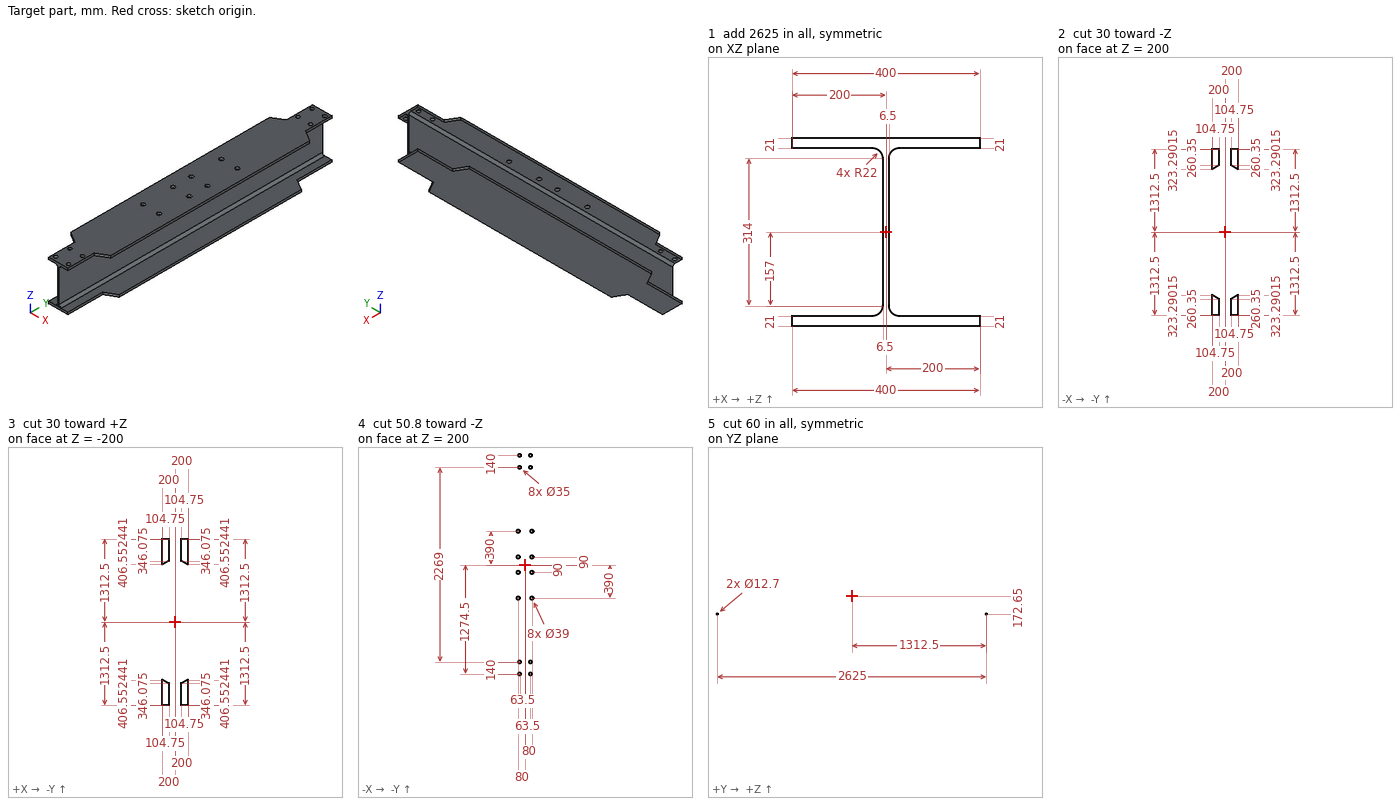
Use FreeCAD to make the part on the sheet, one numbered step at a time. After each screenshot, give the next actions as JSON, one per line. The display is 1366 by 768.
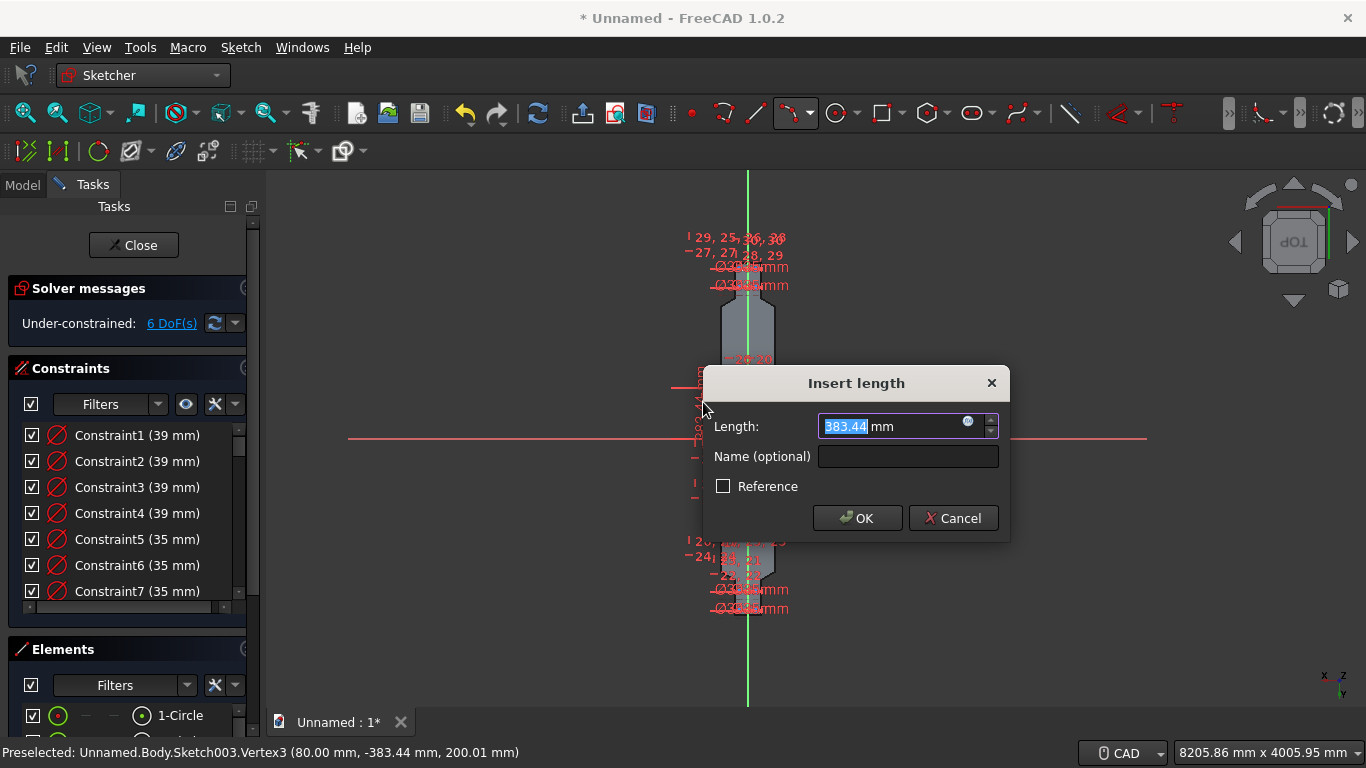
{"action": "type", "text": "390"}
{"action": "key", "text": "Return"}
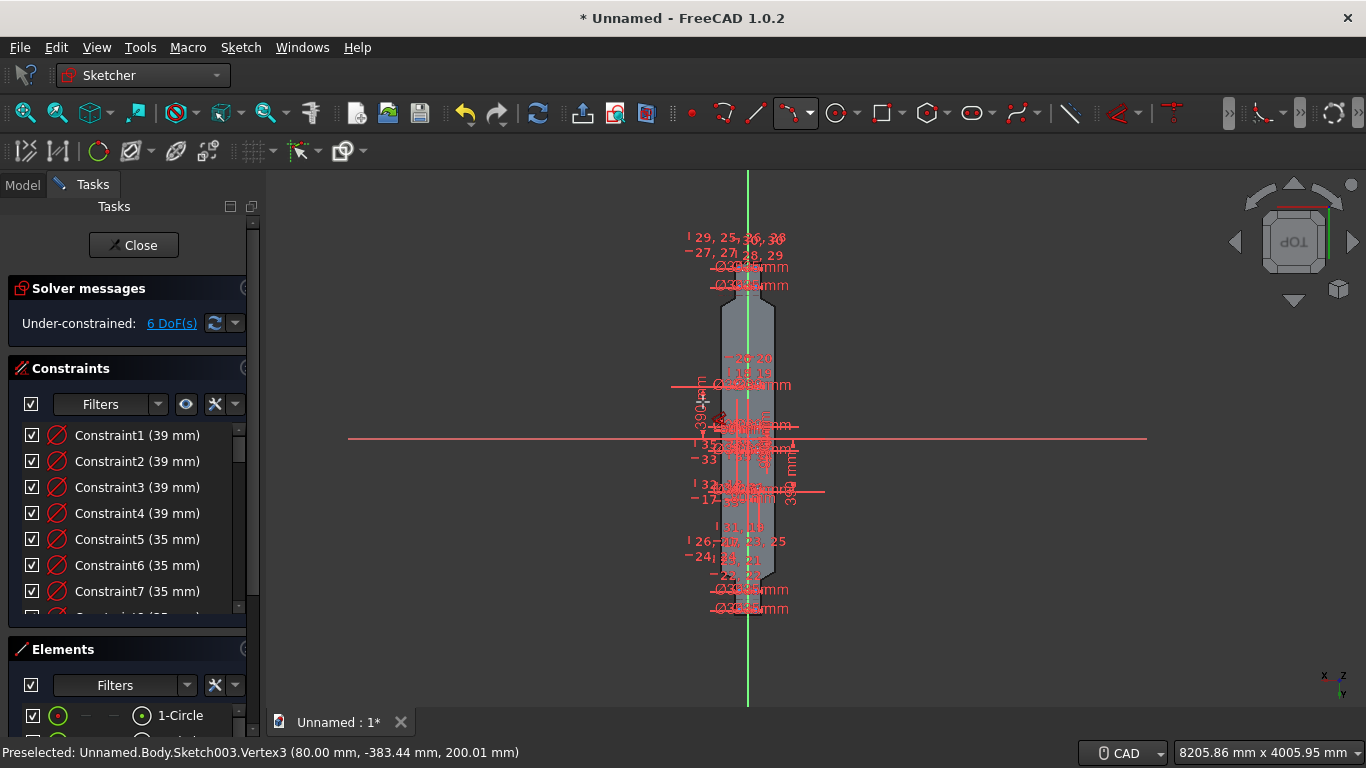
{"action": "scroll", "coordinate": [740, 611], "scroll_direction": "up", "scroll_amount": 8}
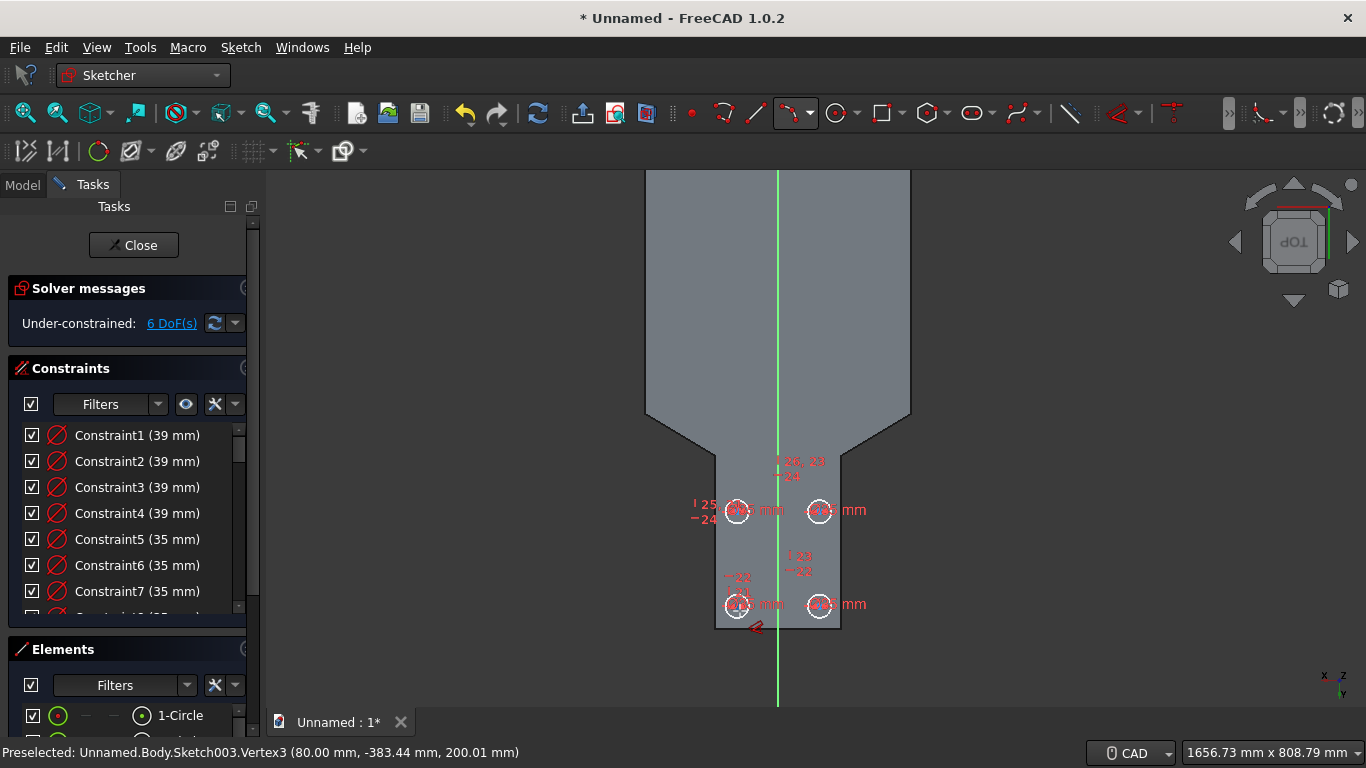
{"action": "left_click", "coordinate": [737, 606]}
{"action": "left_click", "coordinate": [758, 640]}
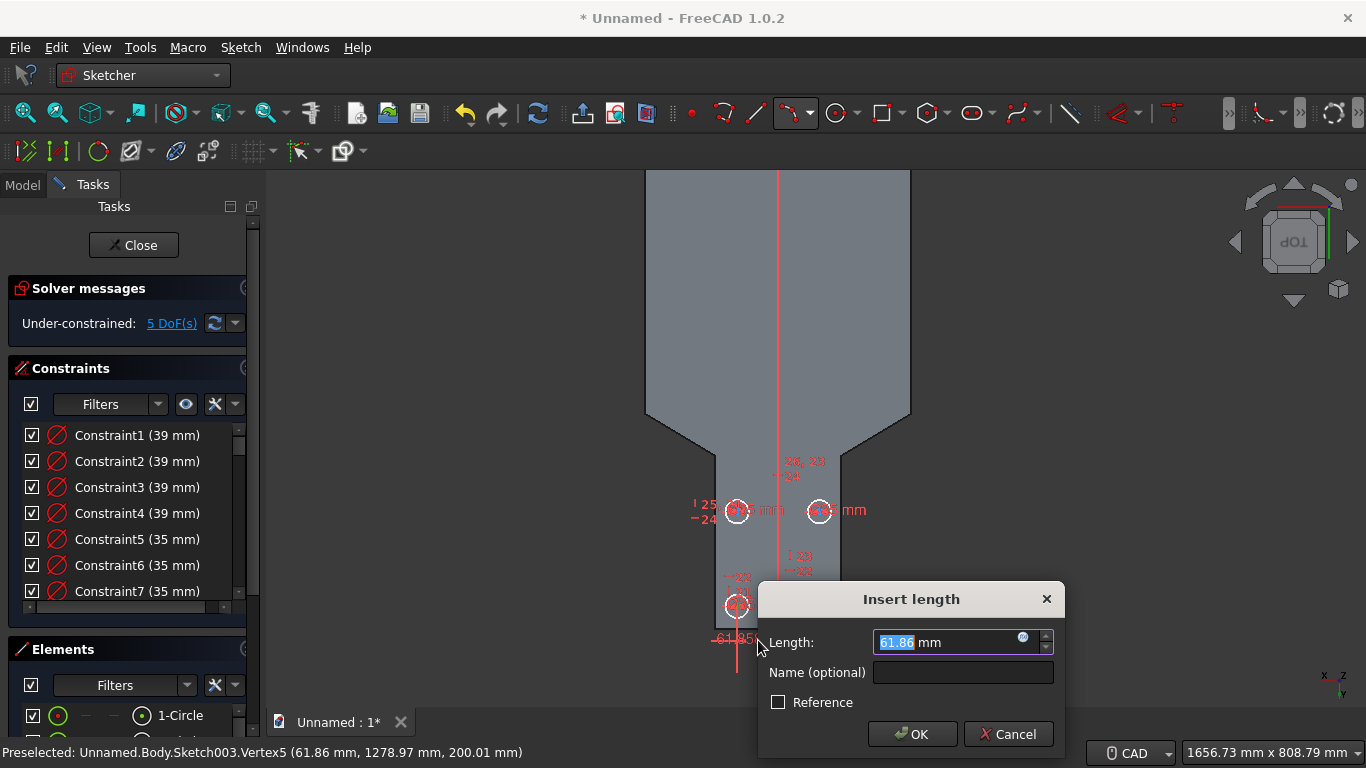
{"action": "type", "text": "63.5"}
{"action": "key", "text": "Return"}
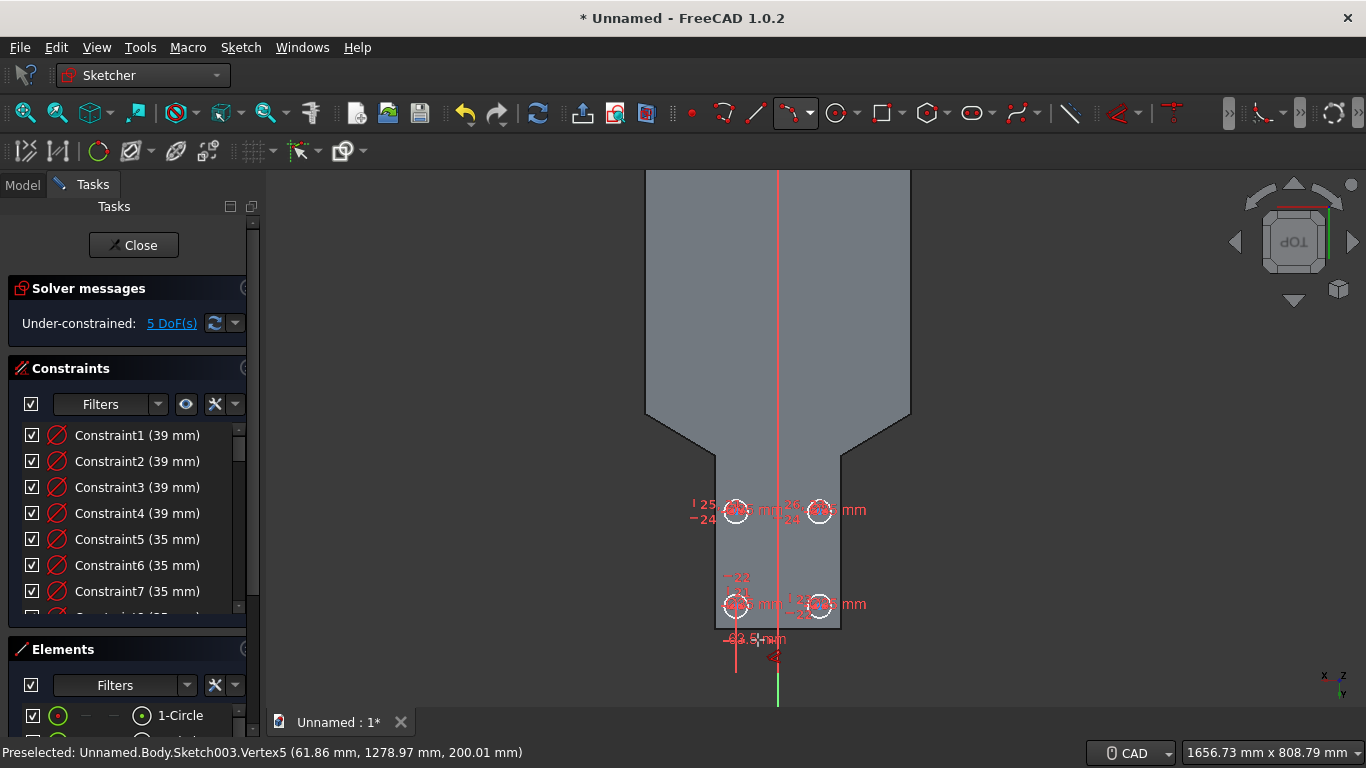
{"action": "left_click", "coordinate": [820, 606]}
{"action": "left_click", "coordinate": [799, 664]}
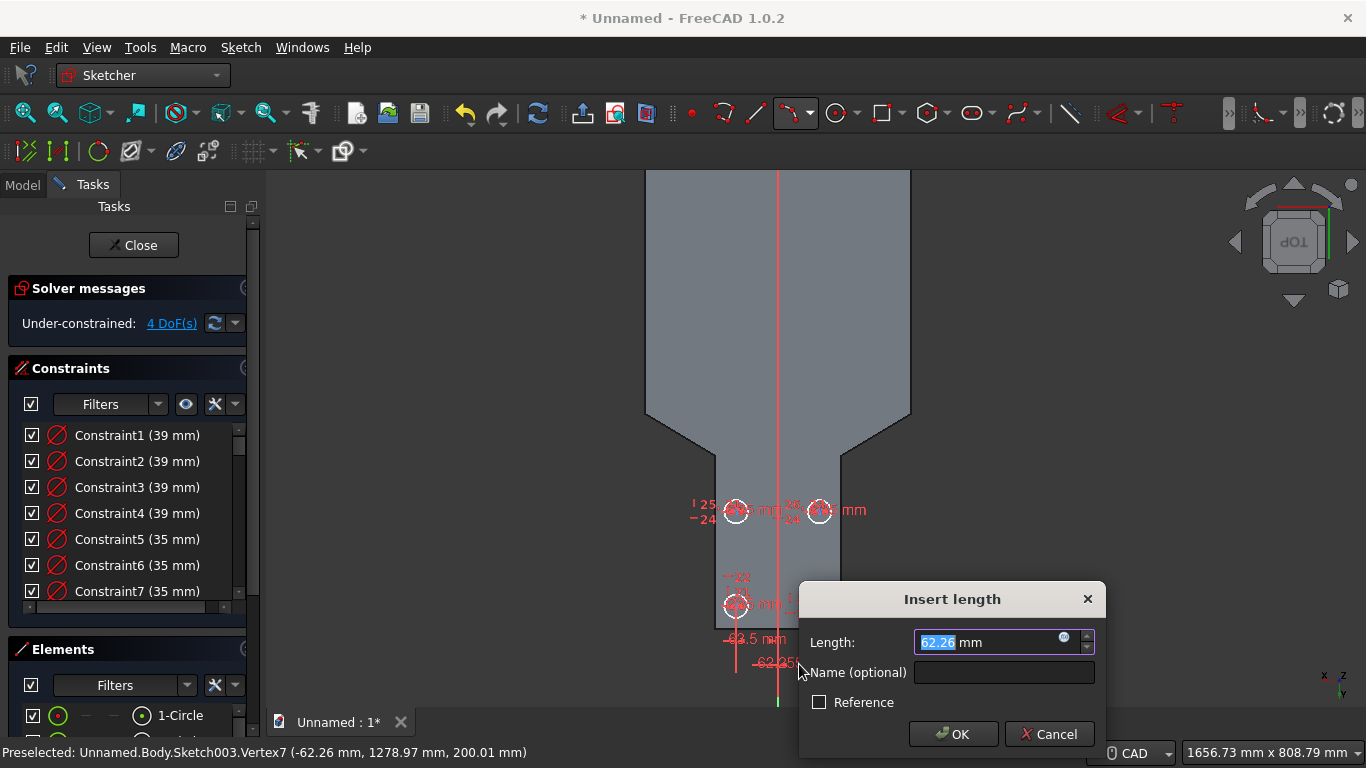
{"action": "type", "text": "63.5"}
{"action": "key", "text": "Return"}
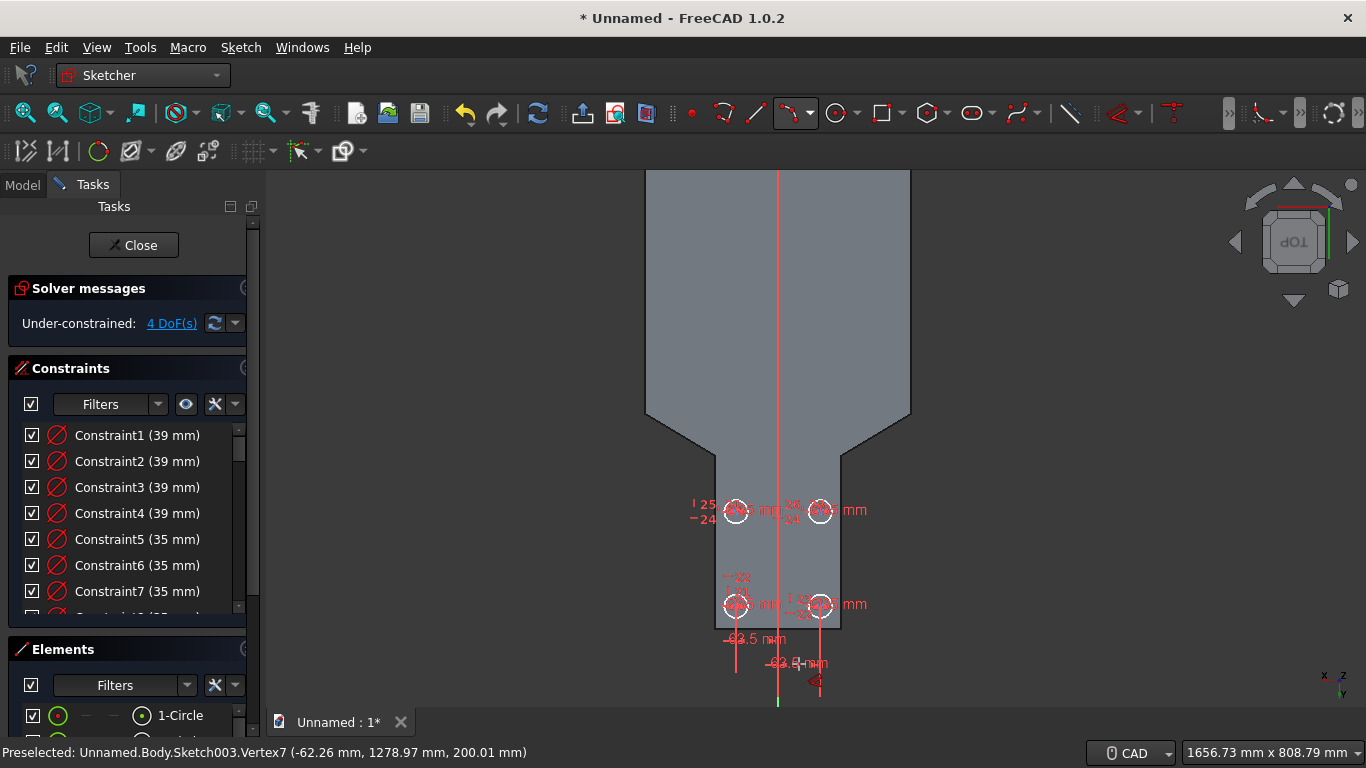
{"action": "left_click", "coordinate": [736, 606]}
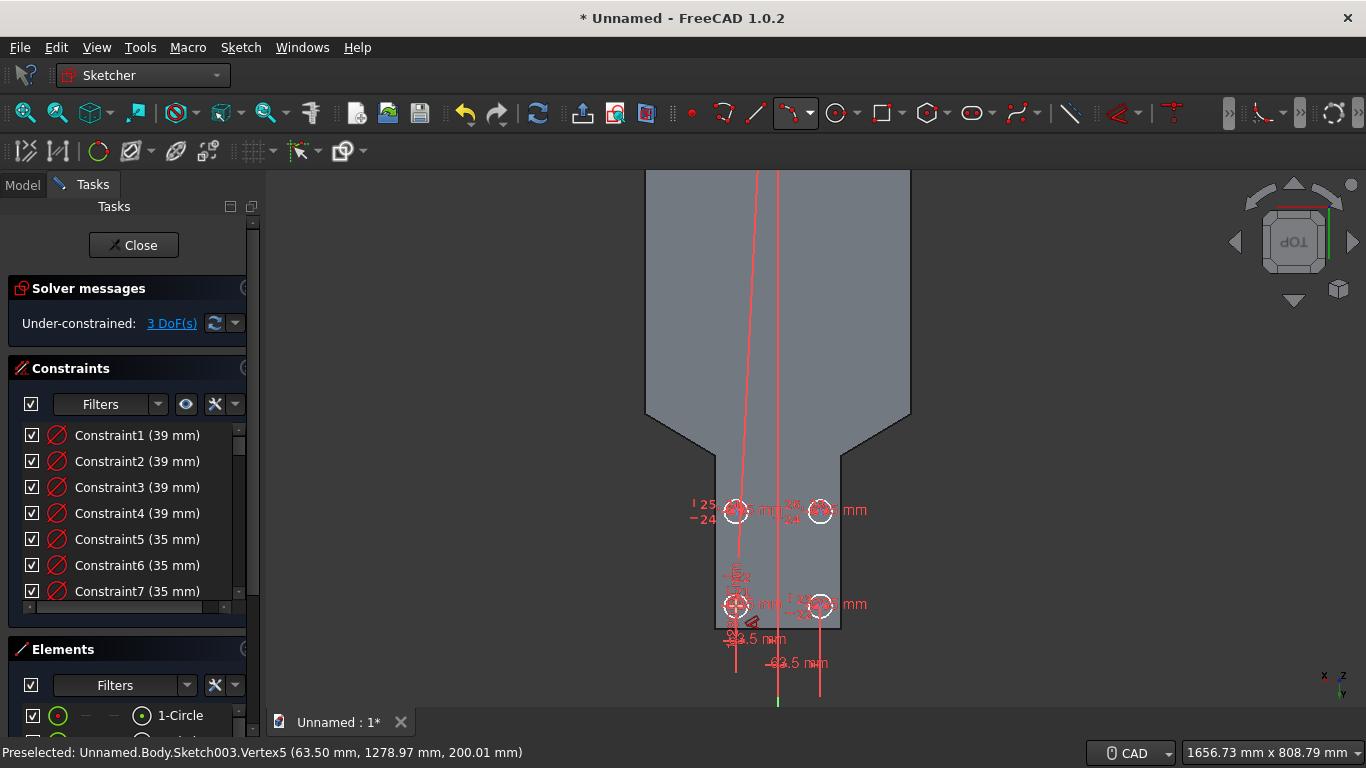
{"action": "left_click", "coordinate": [736, 512]}
{"action": "left_click", "coordinate": [702, 559]}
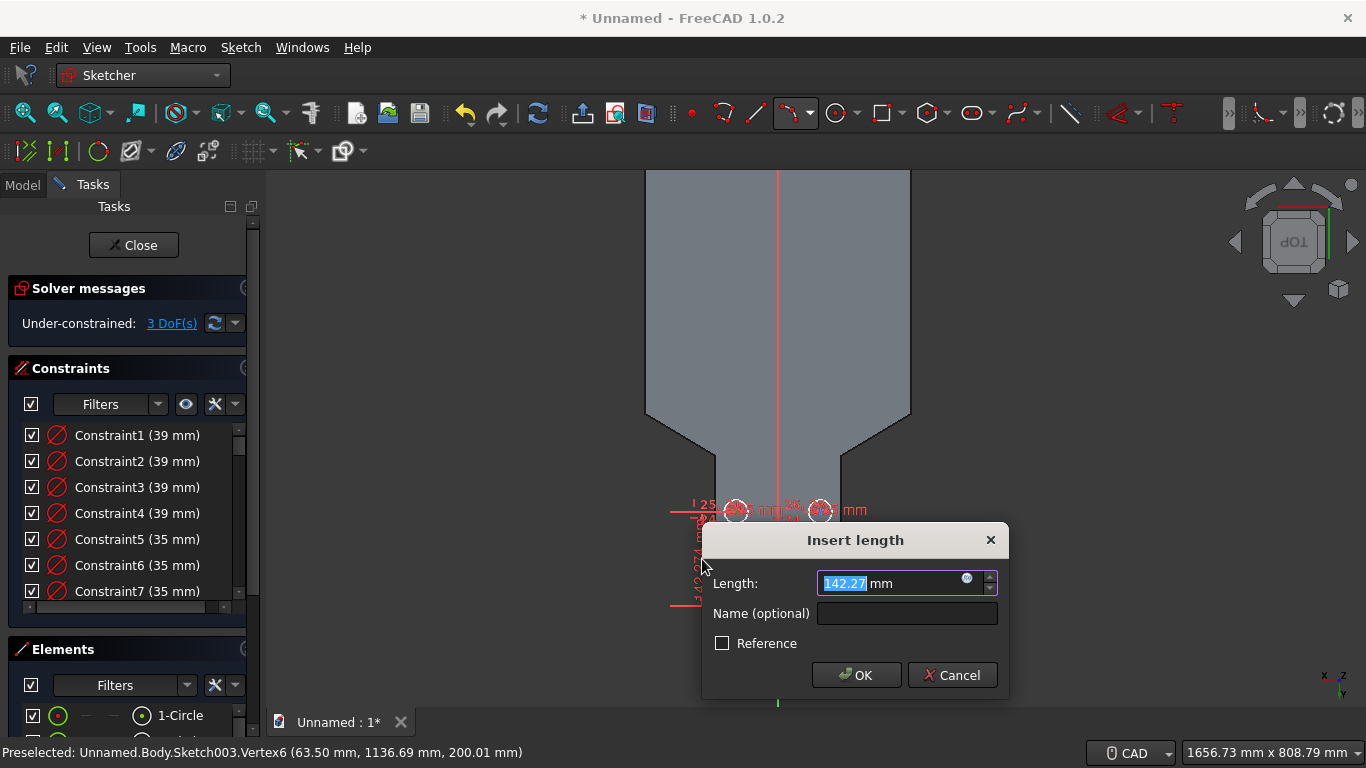
{"action": "type", "text": "140"}
{"action": "key", "text": "Return"}